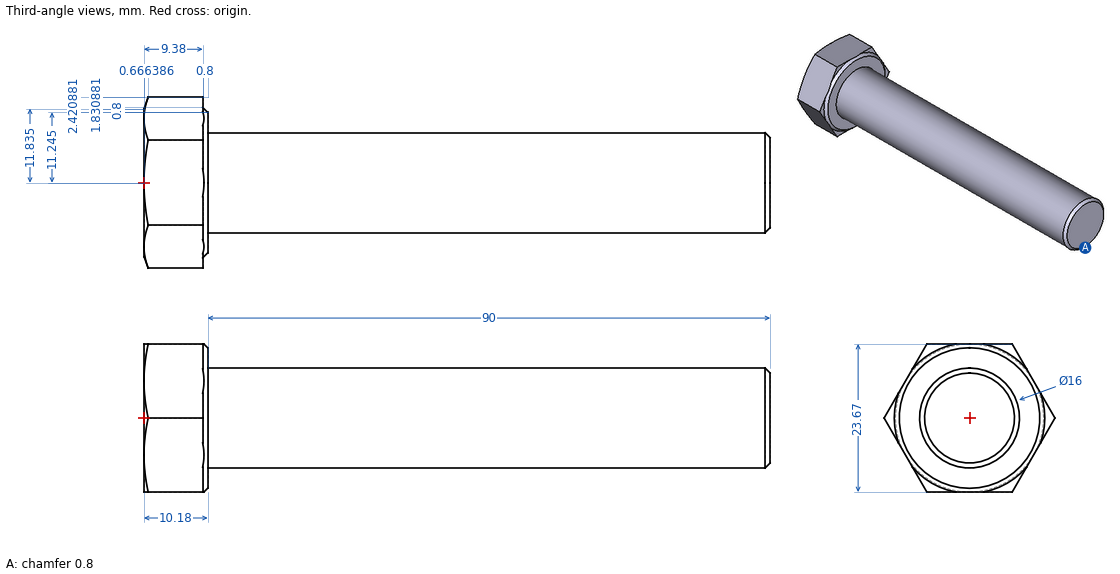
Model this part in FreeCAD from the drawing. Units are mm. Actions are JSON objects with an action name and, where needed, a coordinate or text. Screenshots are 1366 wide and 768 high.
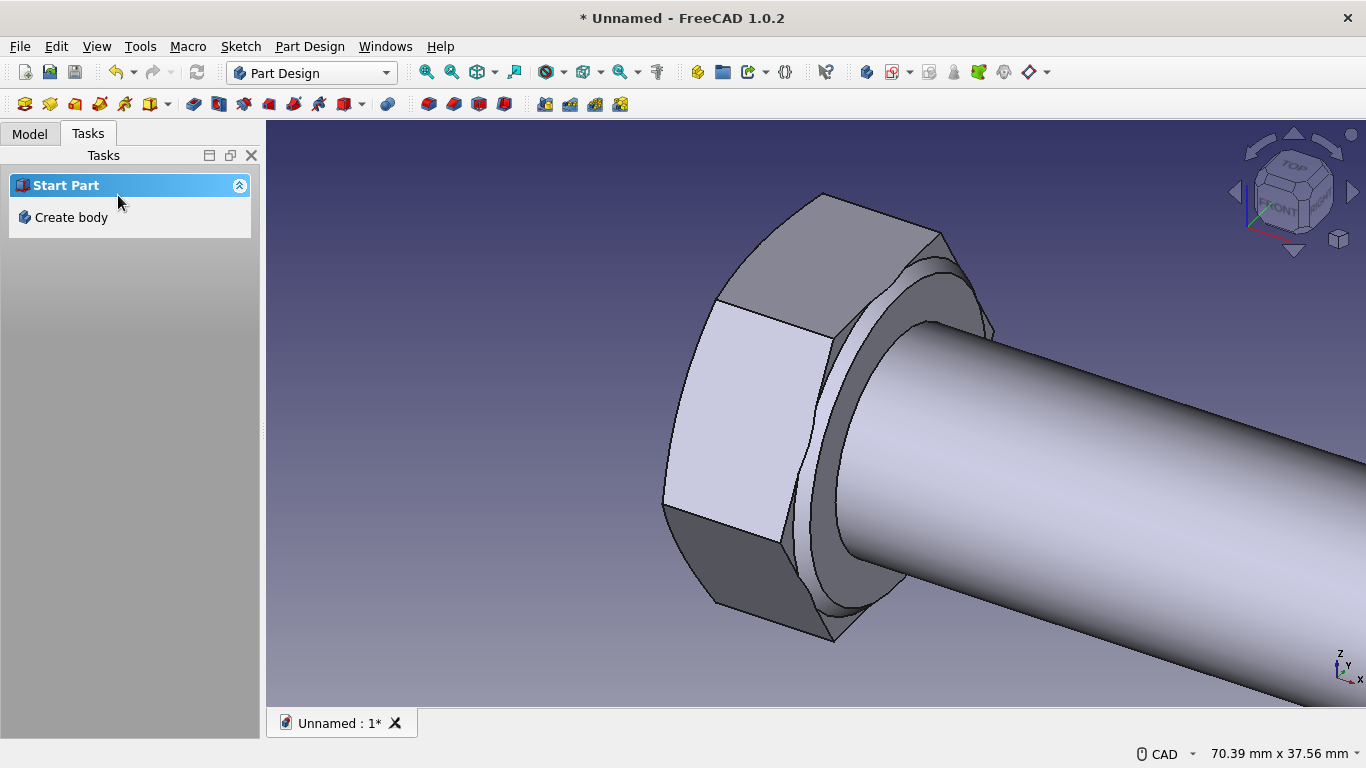
{"action": "key", "text": "v f"}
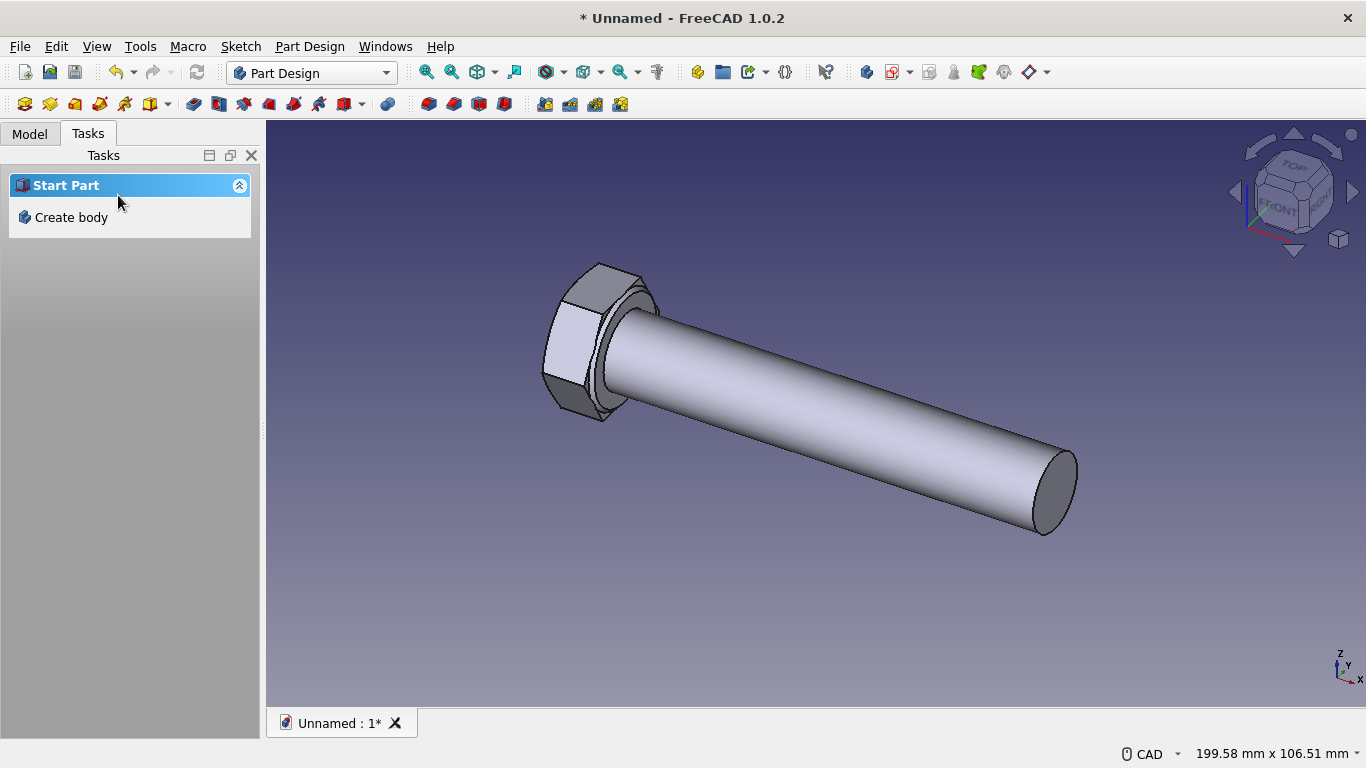
{"action": "left_click", "coordinate": [1033, 514]}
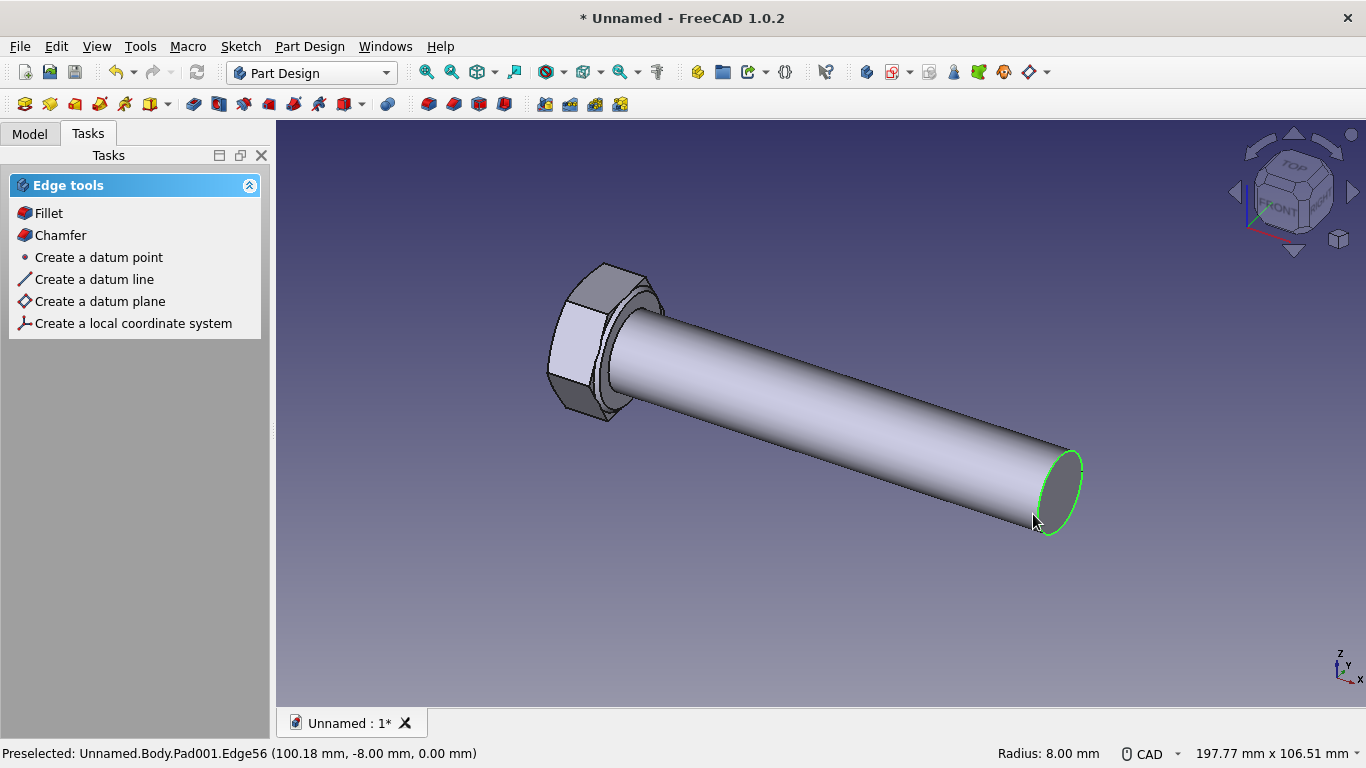
{"action": "left_click", "coordinate": [454, 104]}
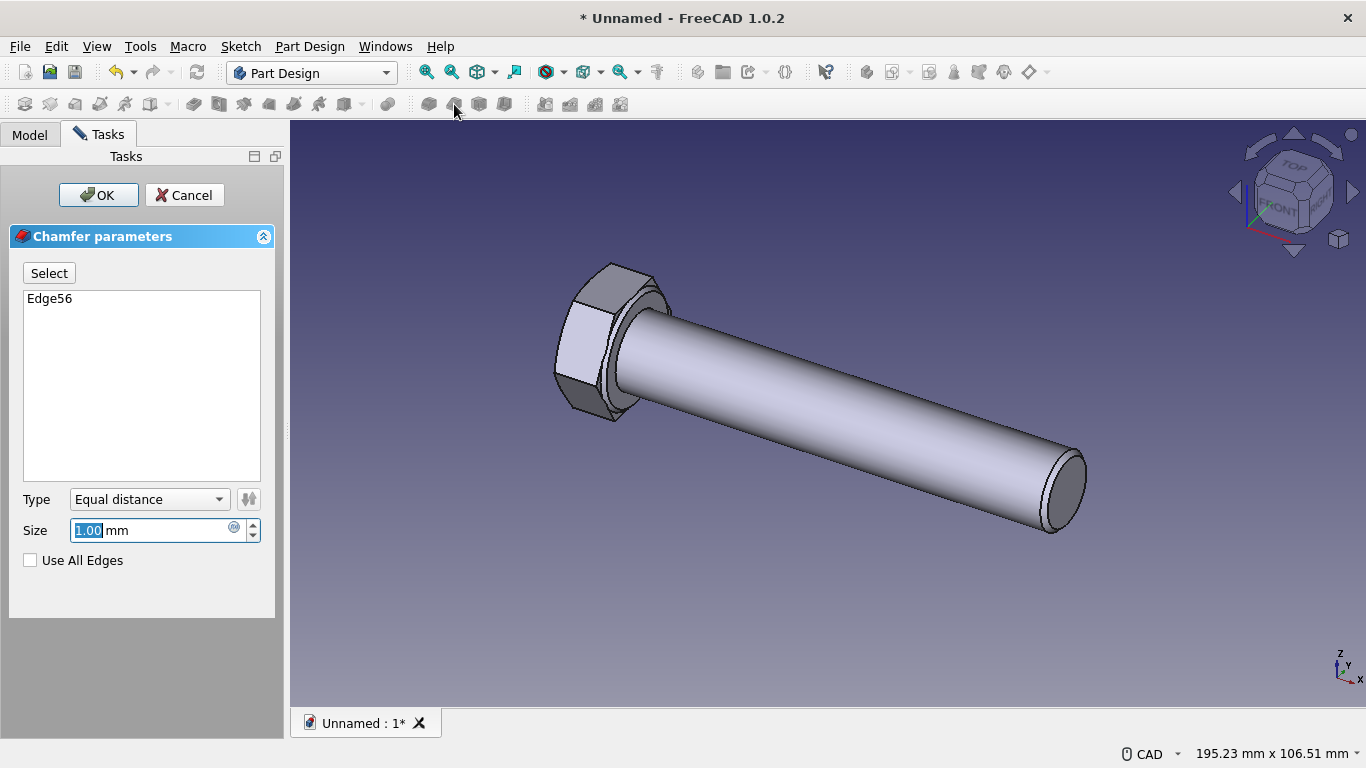
{"action": "type", "text": "0.8"}
{"action": "key", "text": "Tab"}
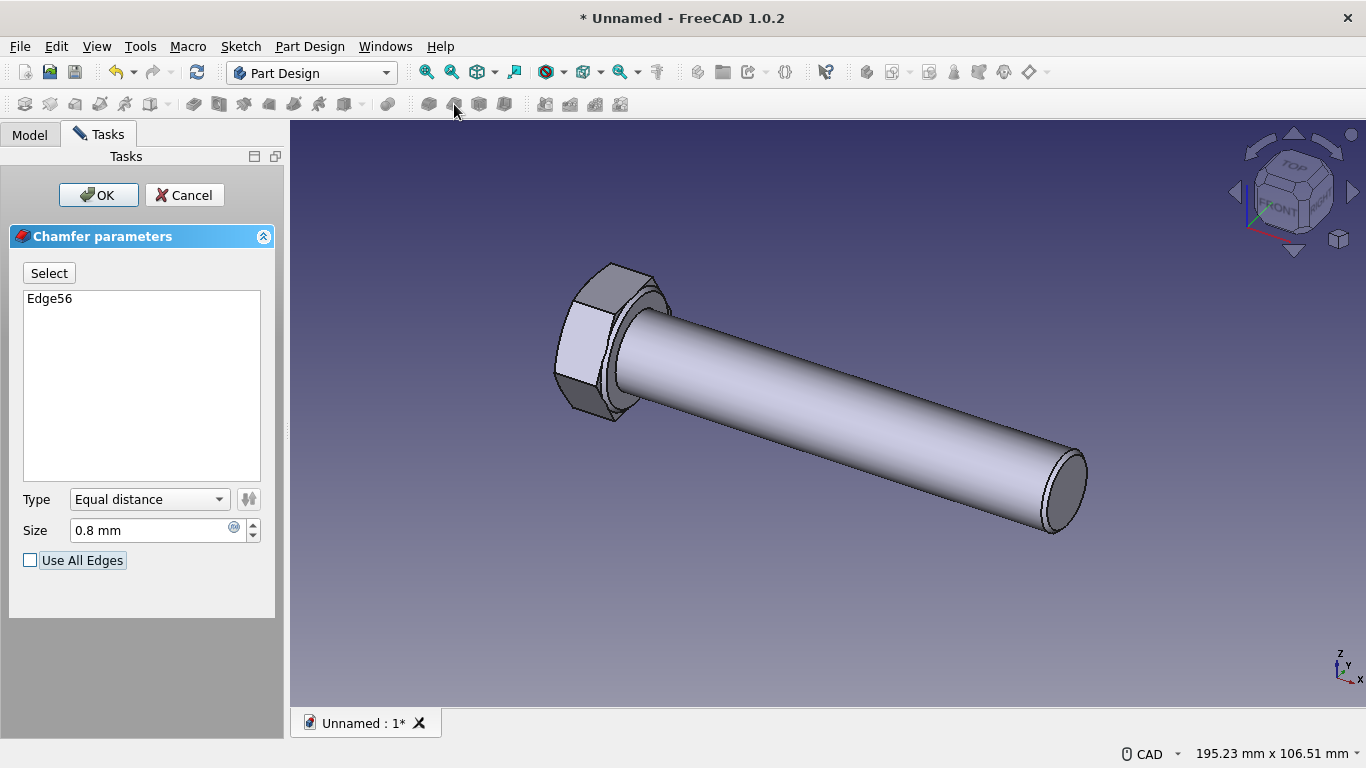
{"action": "left_click", "coordinate": [99, 195]}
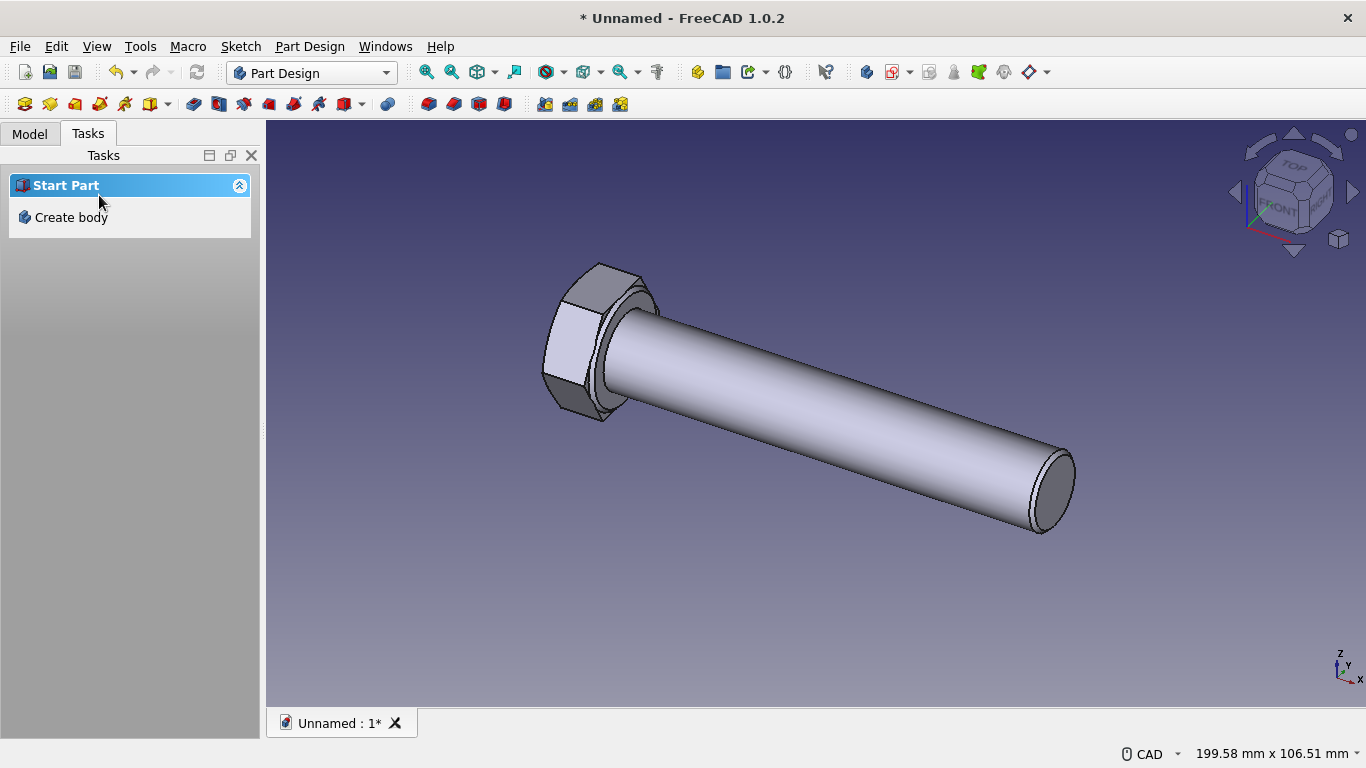
{"action": "key", "text": "0"}